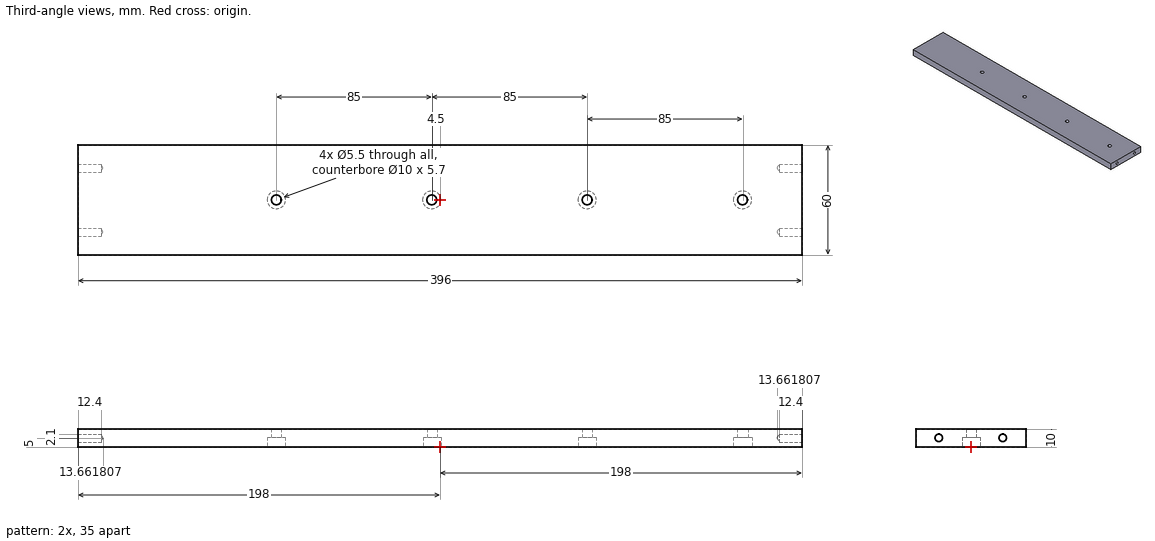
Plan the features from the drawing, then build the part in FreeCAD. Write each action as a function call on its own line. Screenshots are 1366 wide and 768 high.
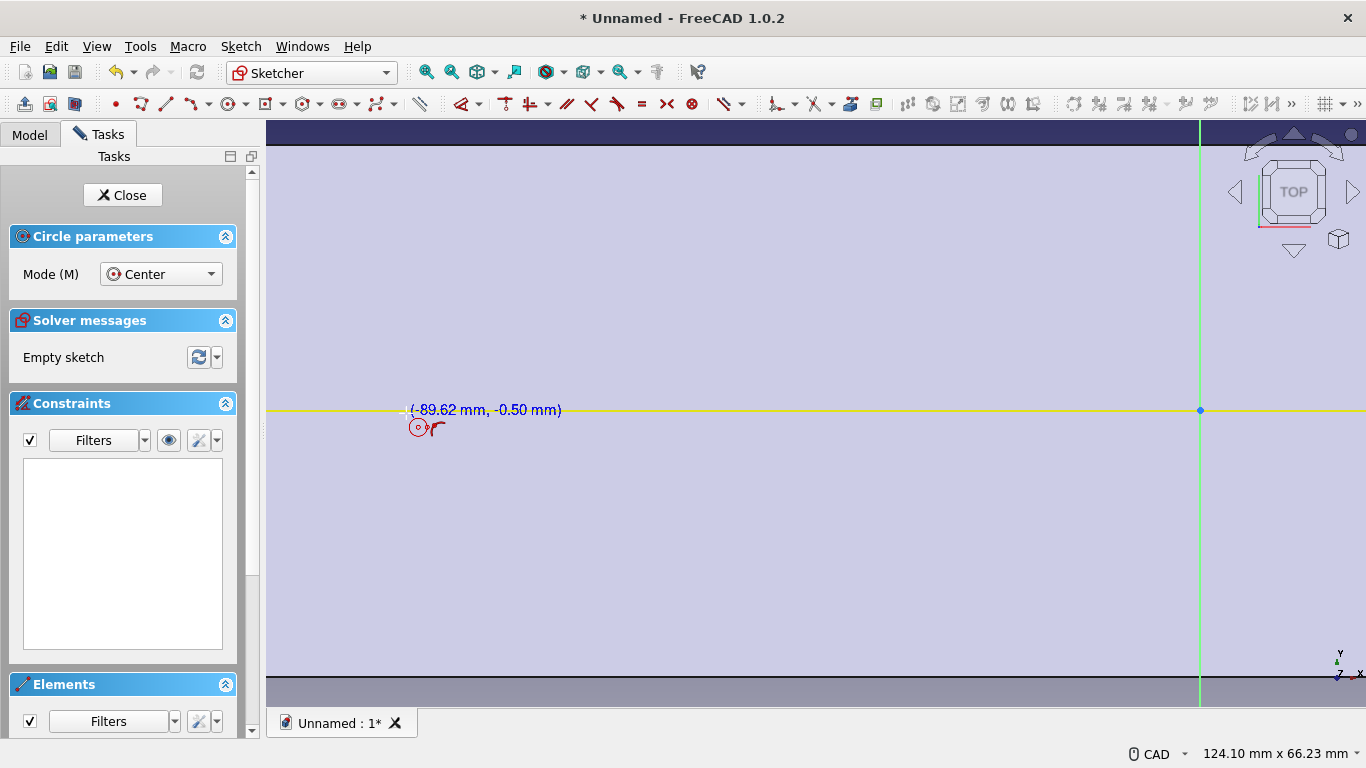
click(407, 411)
move(424, 394)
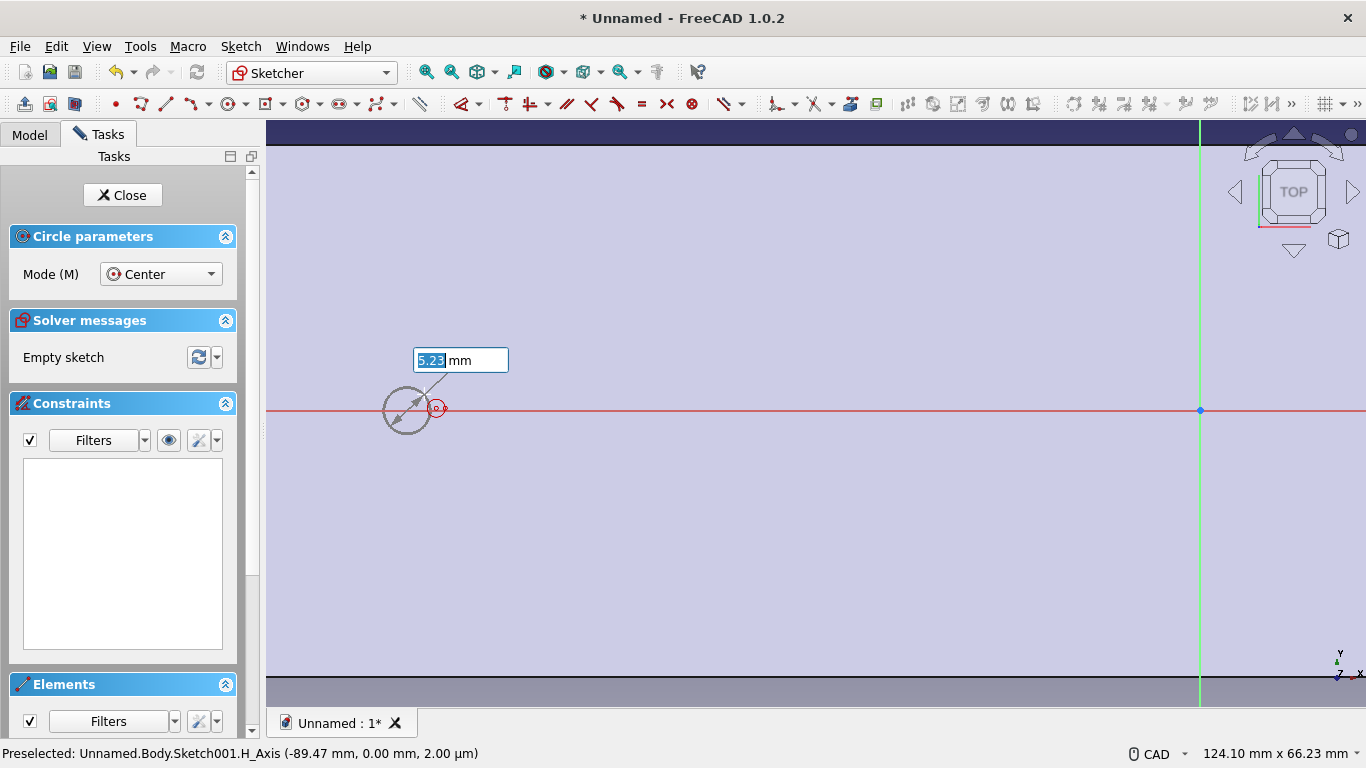
text(5.5)
key(Return)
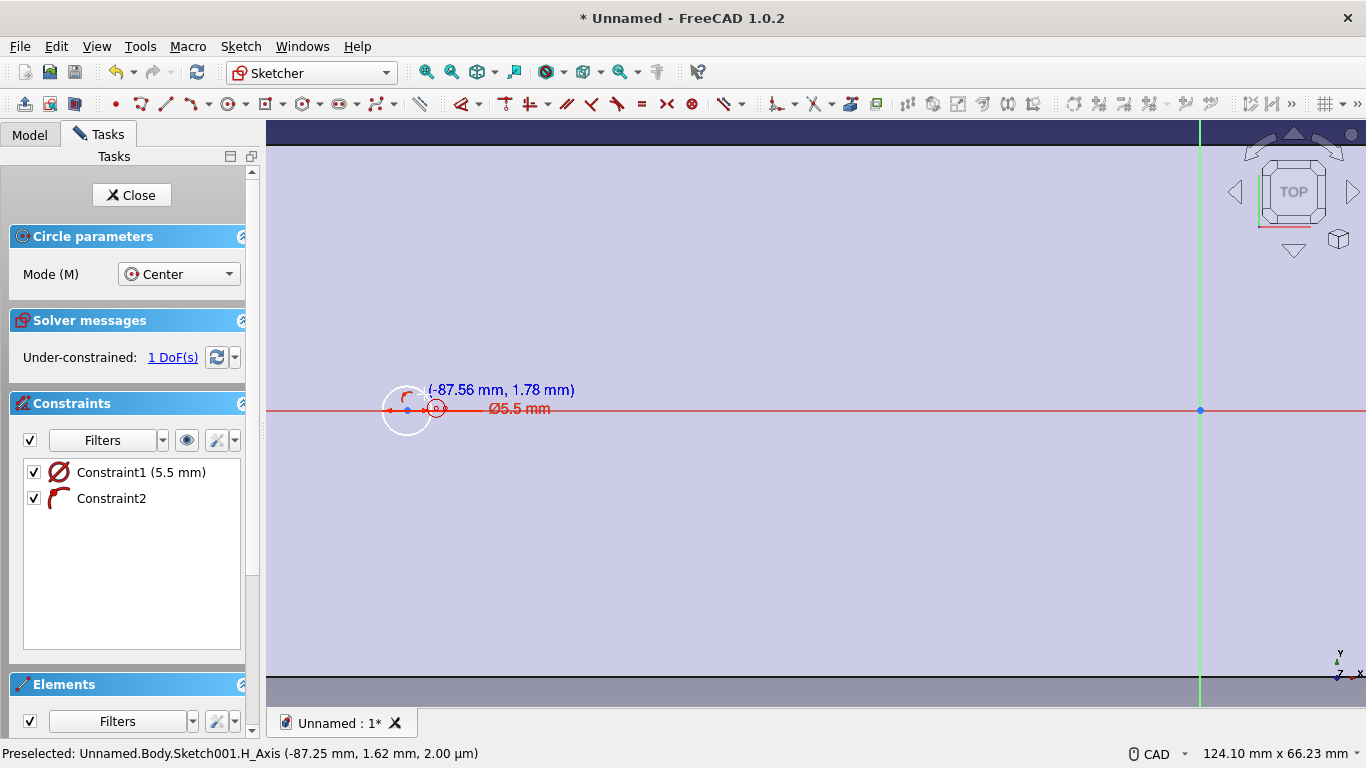
click(1160, 411)
move(1177, 394)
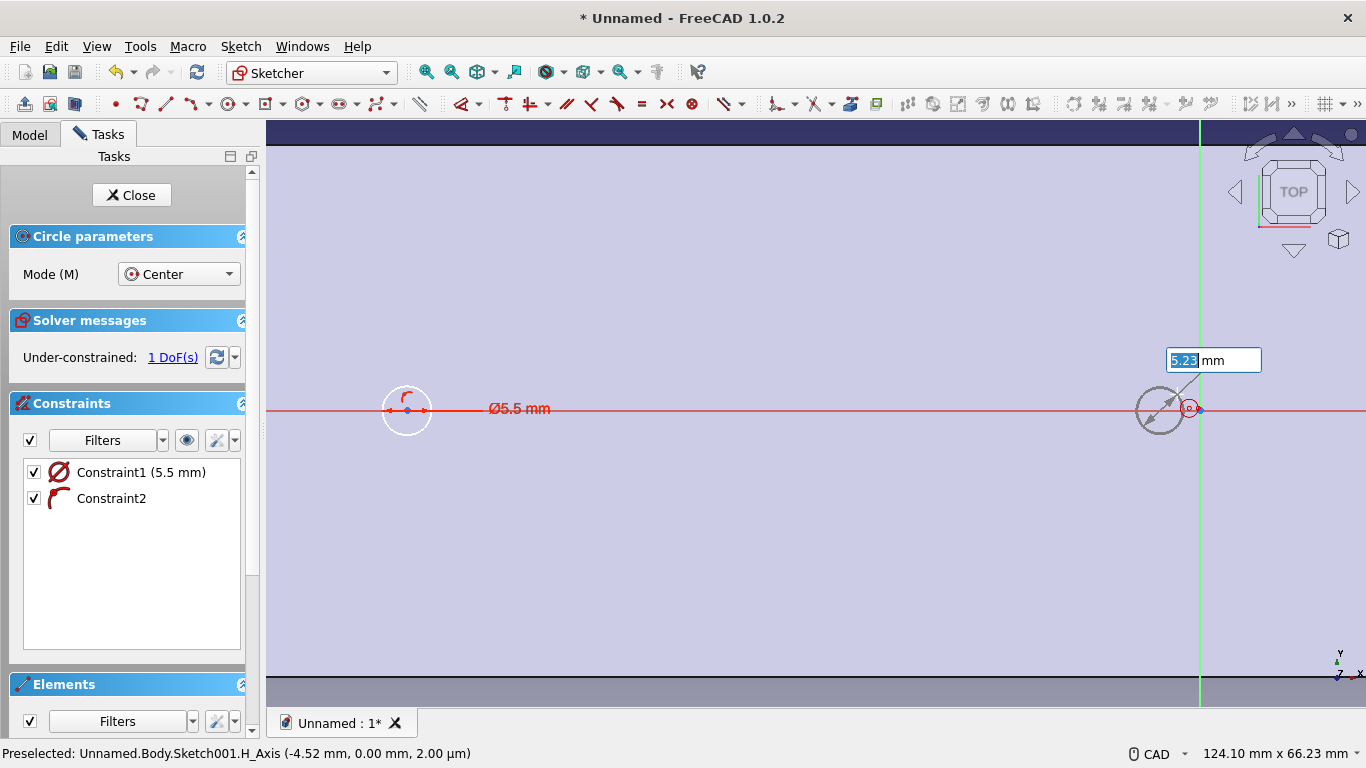
text(5.5)
key(Return)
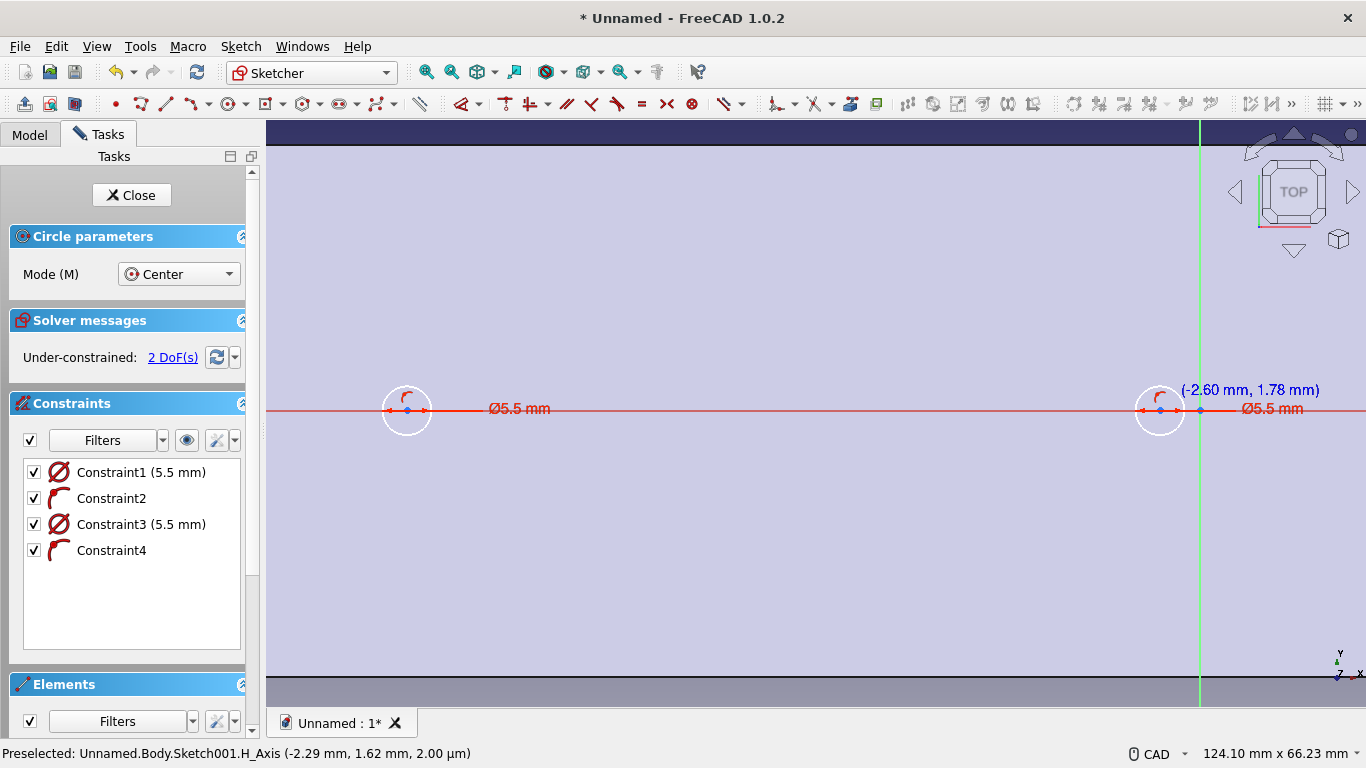
scroll(407, 415, down, 6)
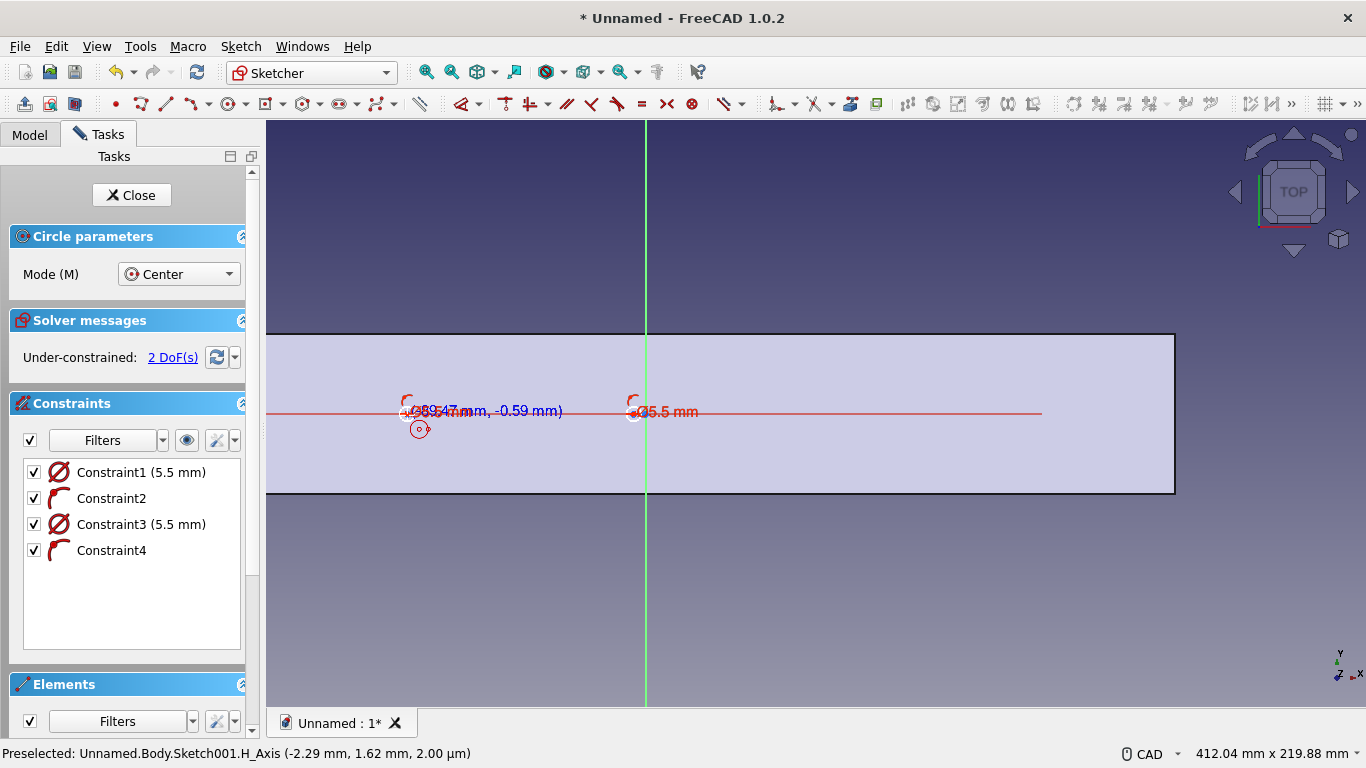
scroll(861, 414, up, 6)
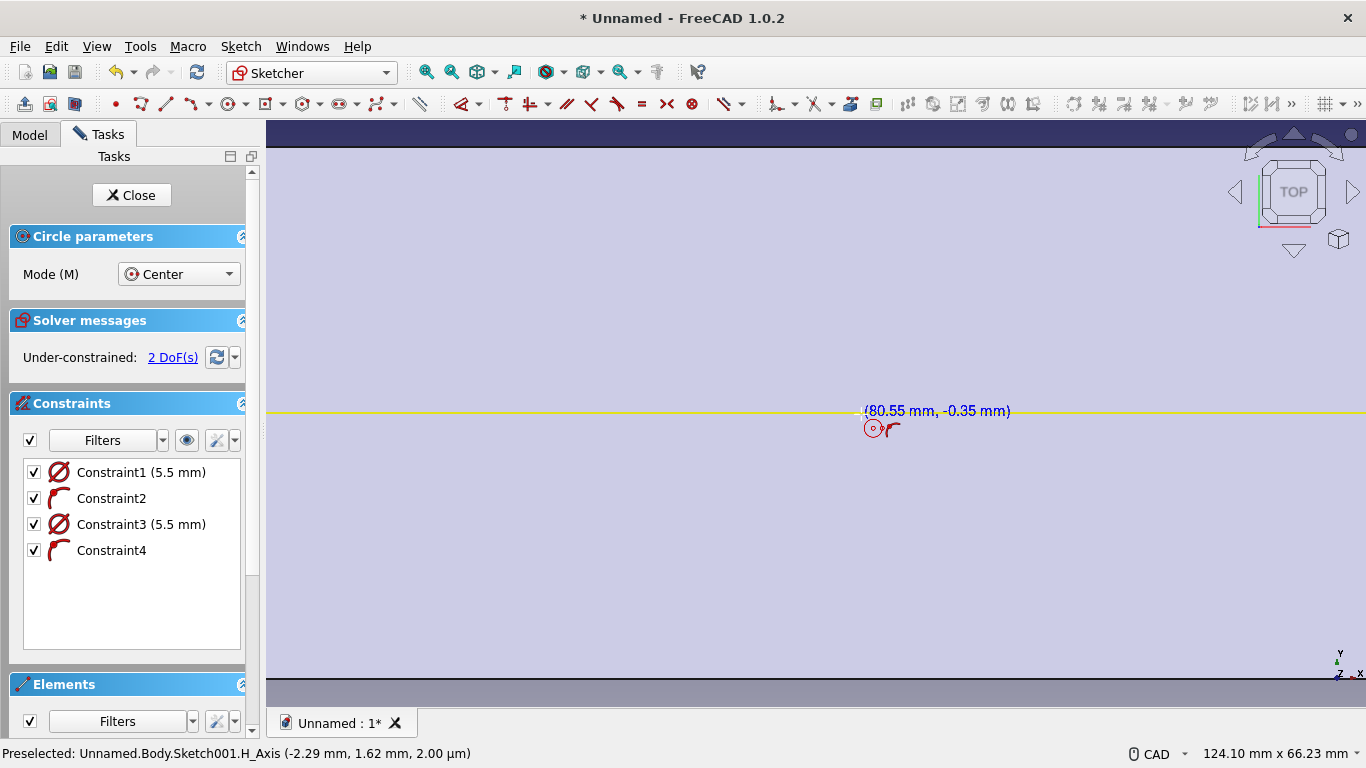
click(859, 413)
move(877, 396)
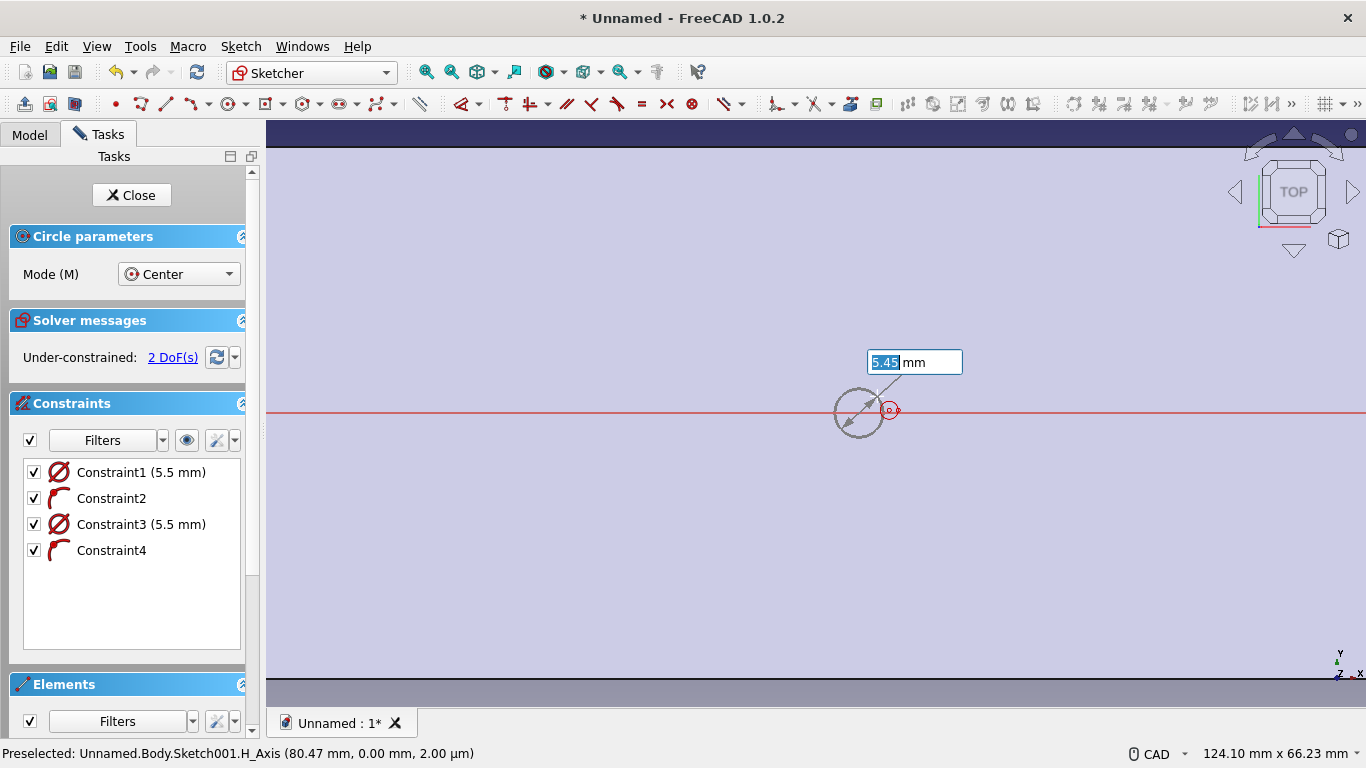
text(5.5)
key(Return)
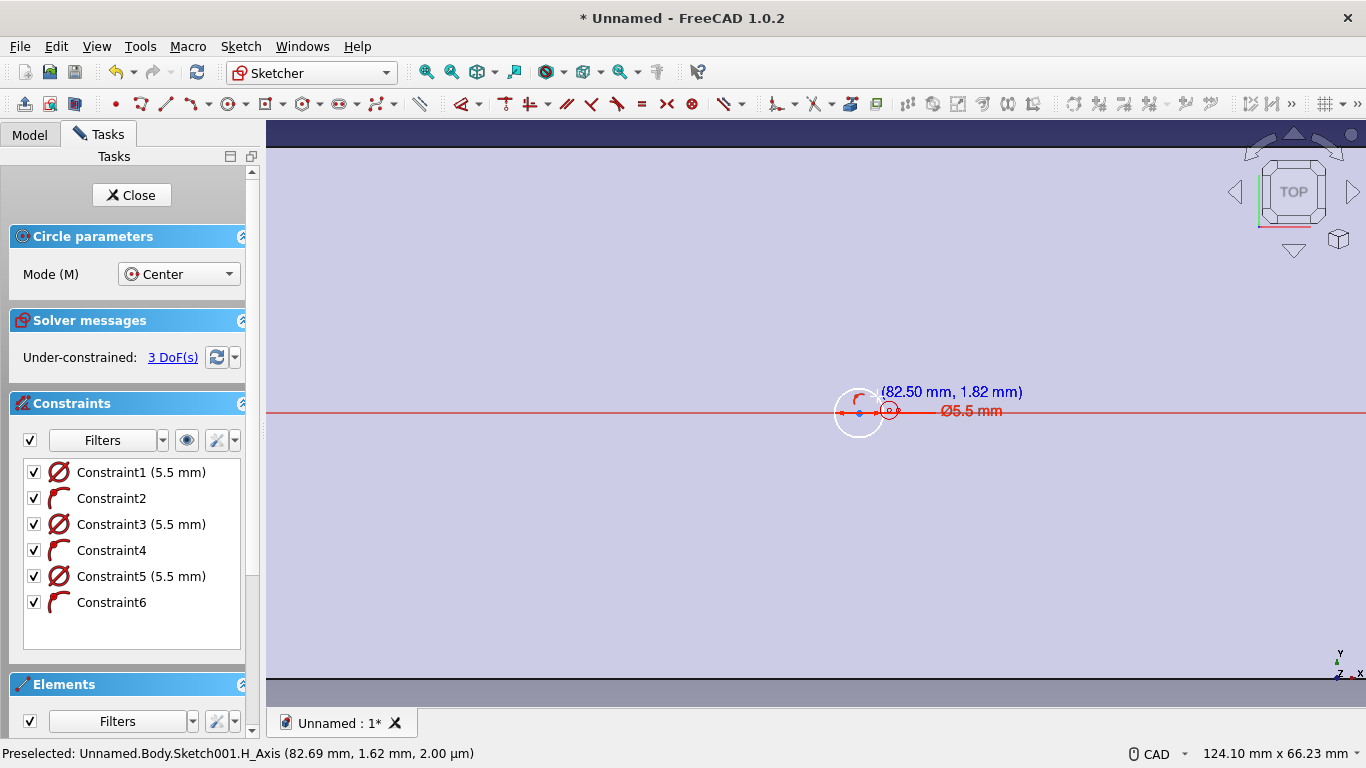
scroll(862, 414, down, 6)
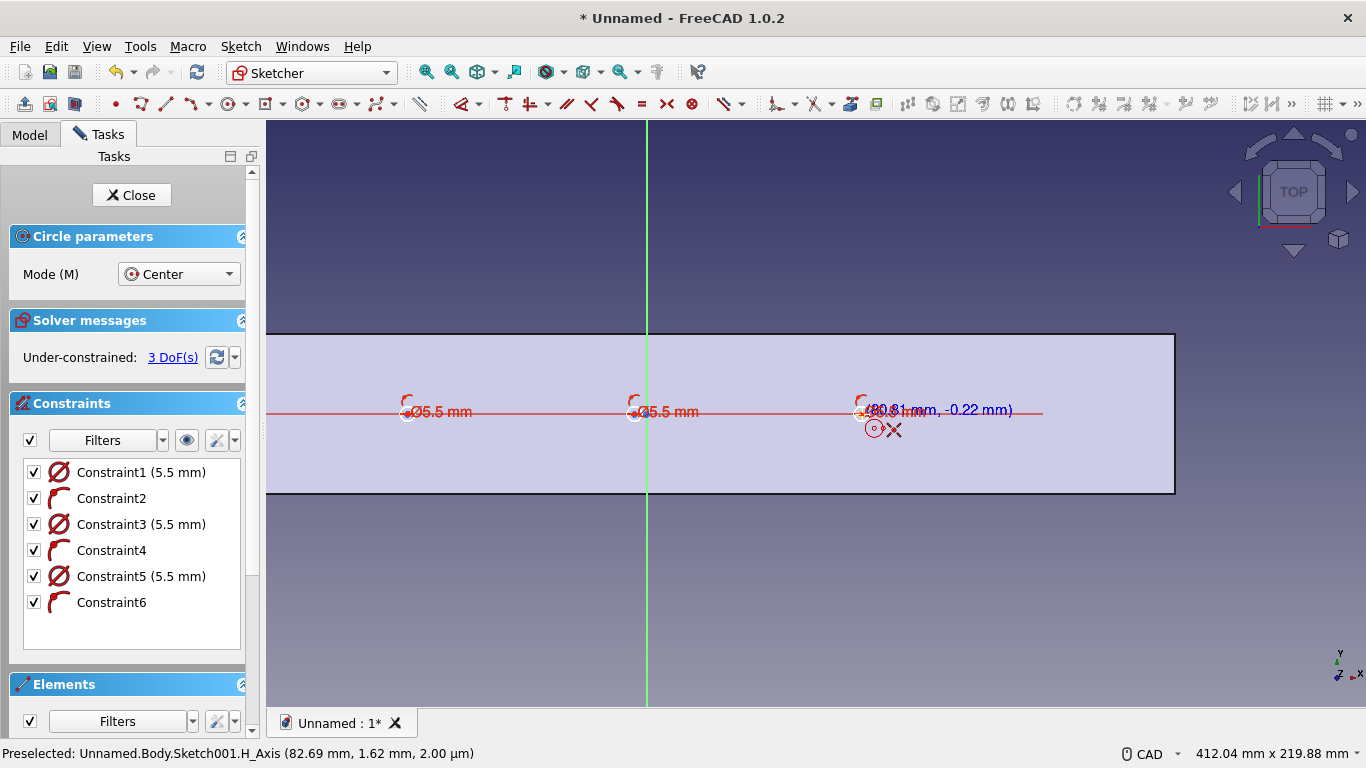
scroll(1088, 414, up, 6)